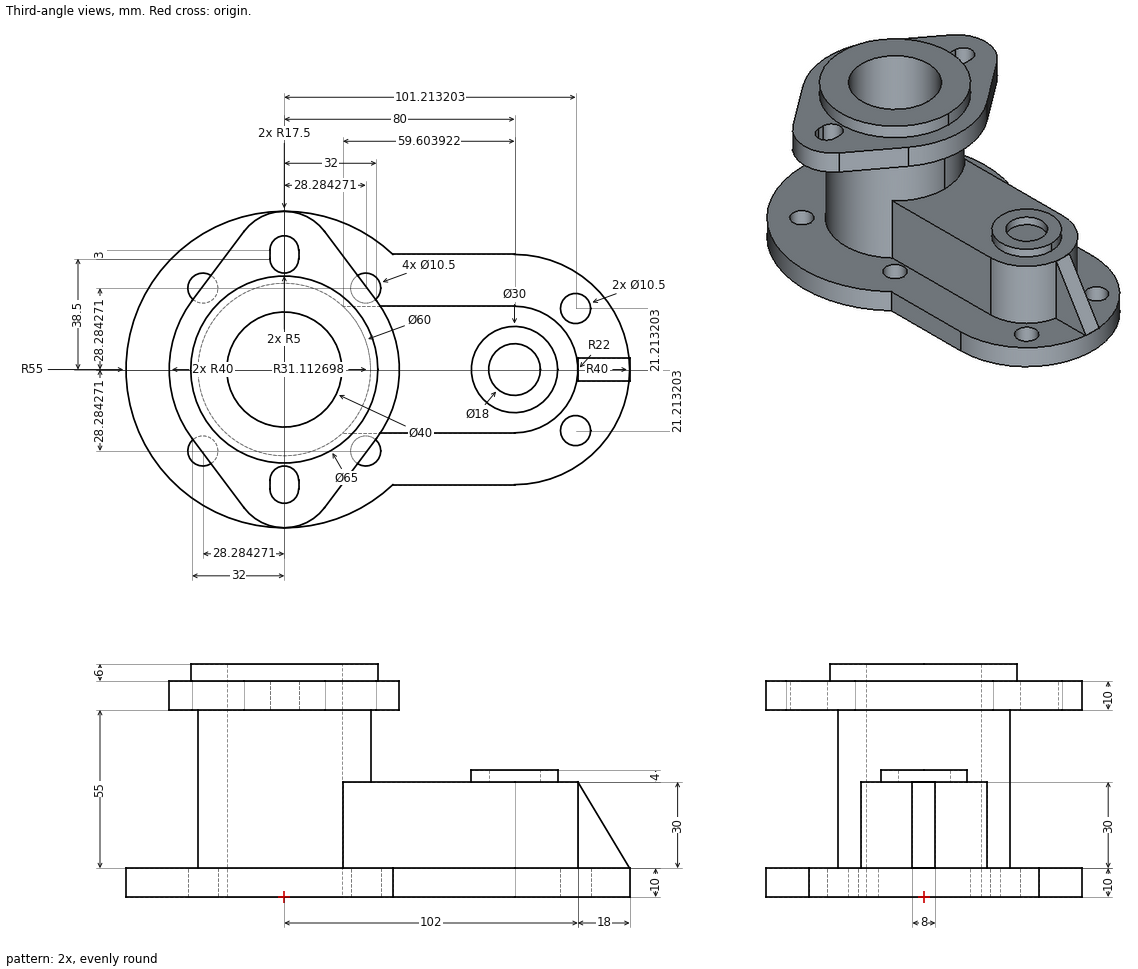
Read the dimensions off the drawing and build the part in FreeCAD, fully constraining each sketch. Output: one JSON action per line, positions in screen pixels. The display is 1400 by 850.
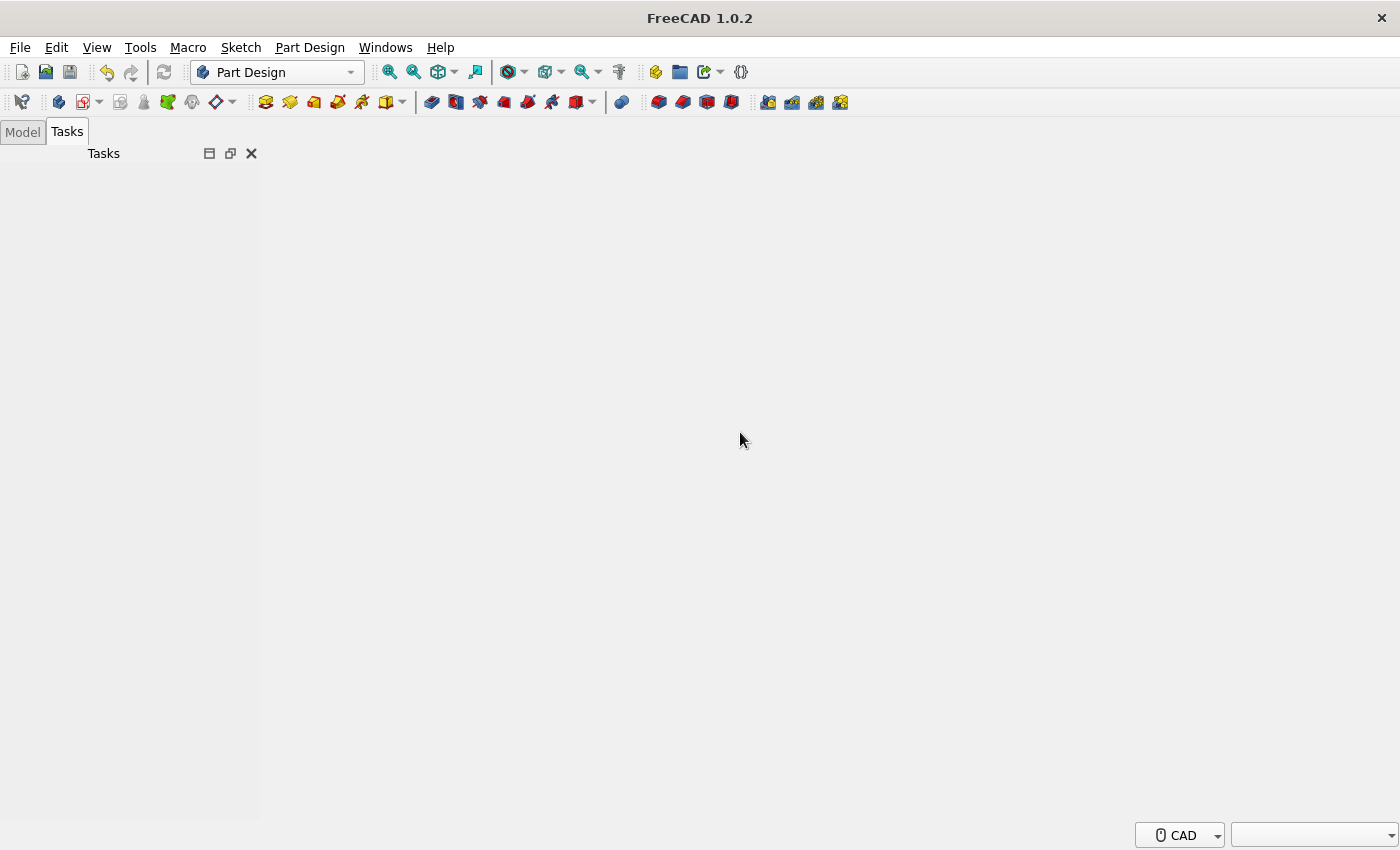
{"action": "key", "text": "ctrl+n"}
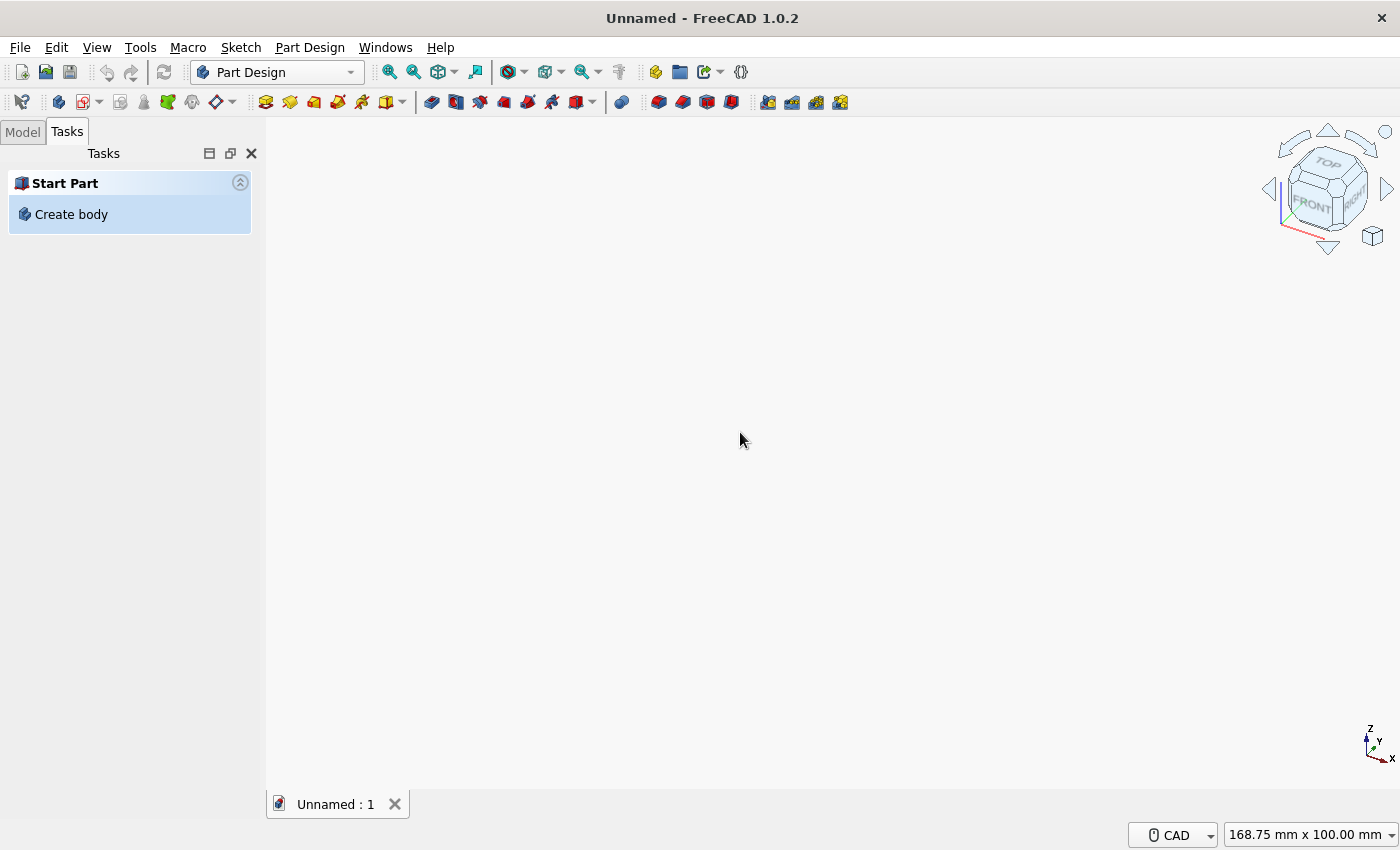
{"action": "left_click", "coordinate": [84, 102]}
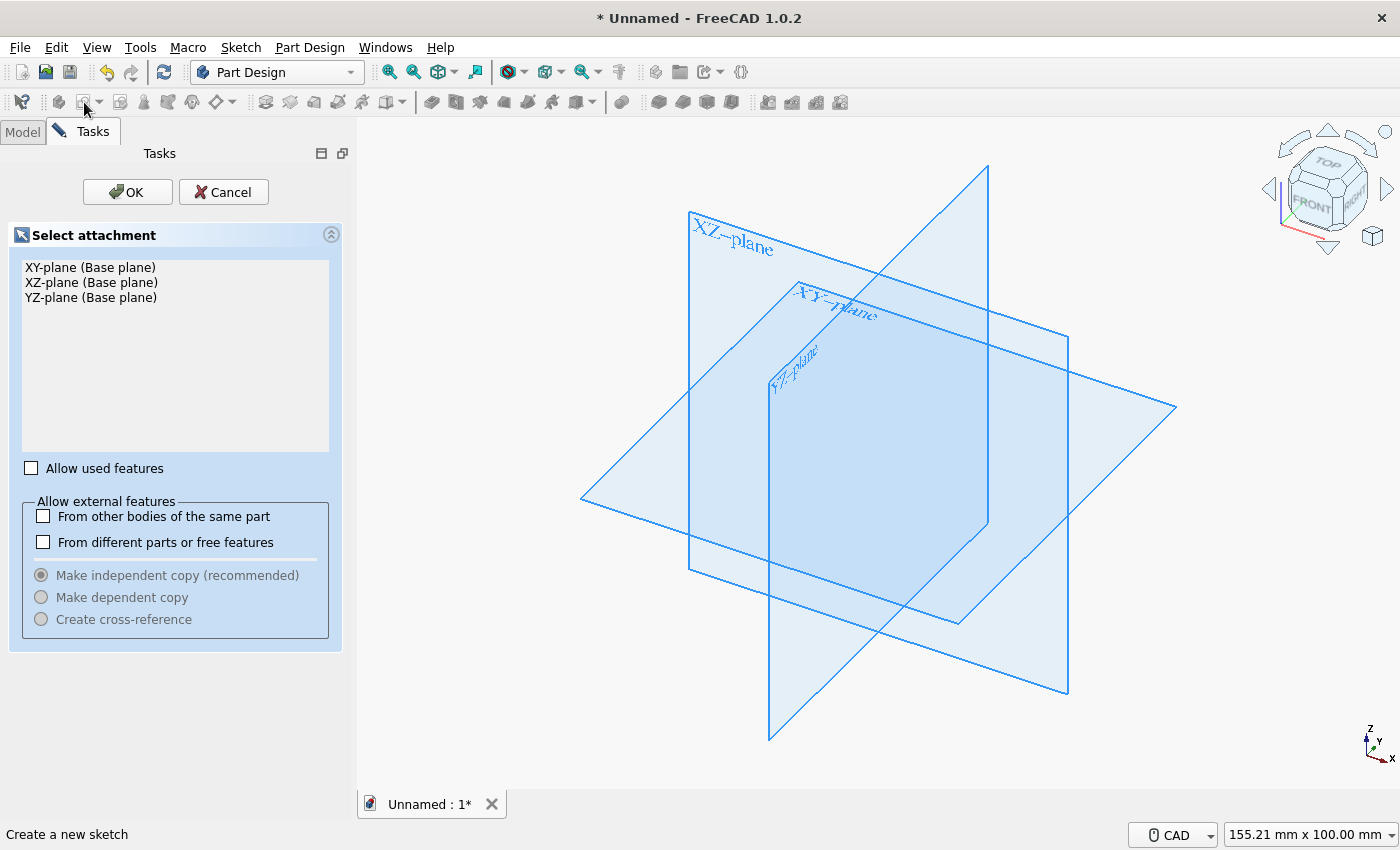
{"action": "left_click", "coordinate": [82, 268]}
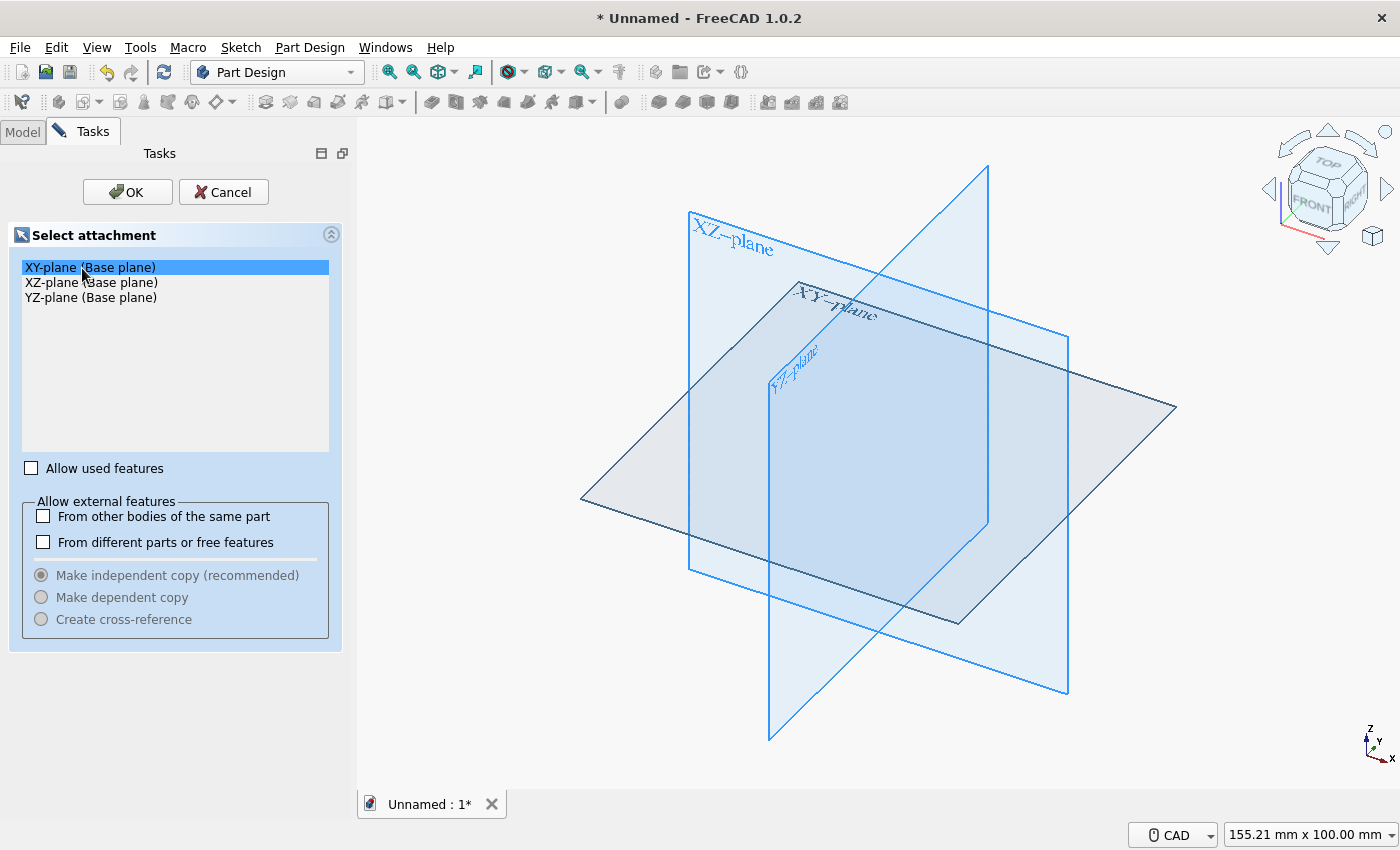
{"action": "left_click", "coordinate": [128, 192]}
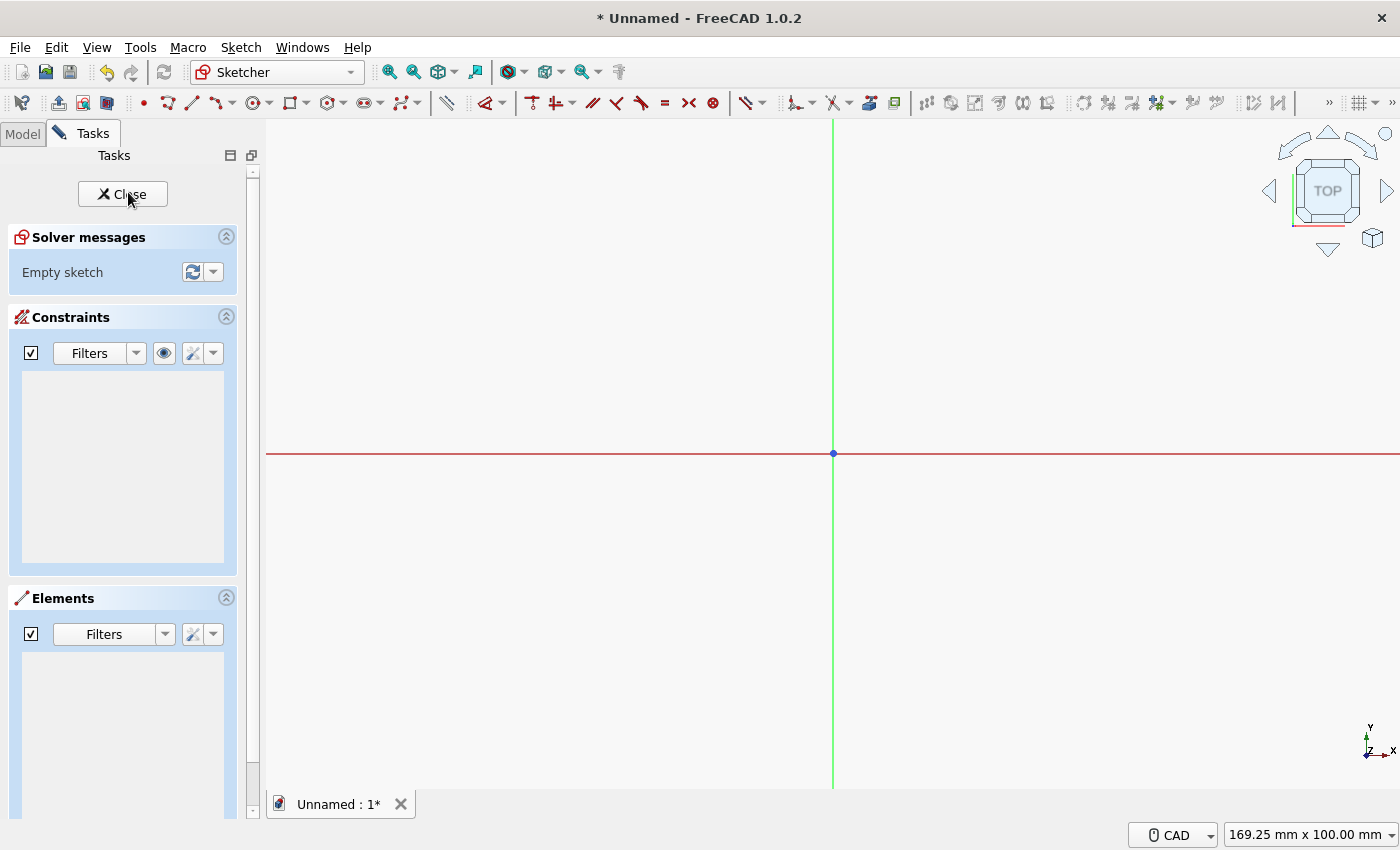
{"action": "scroll", "coordinate": [416, 454], "scroll_direction": "down", "scroll_amount": 3}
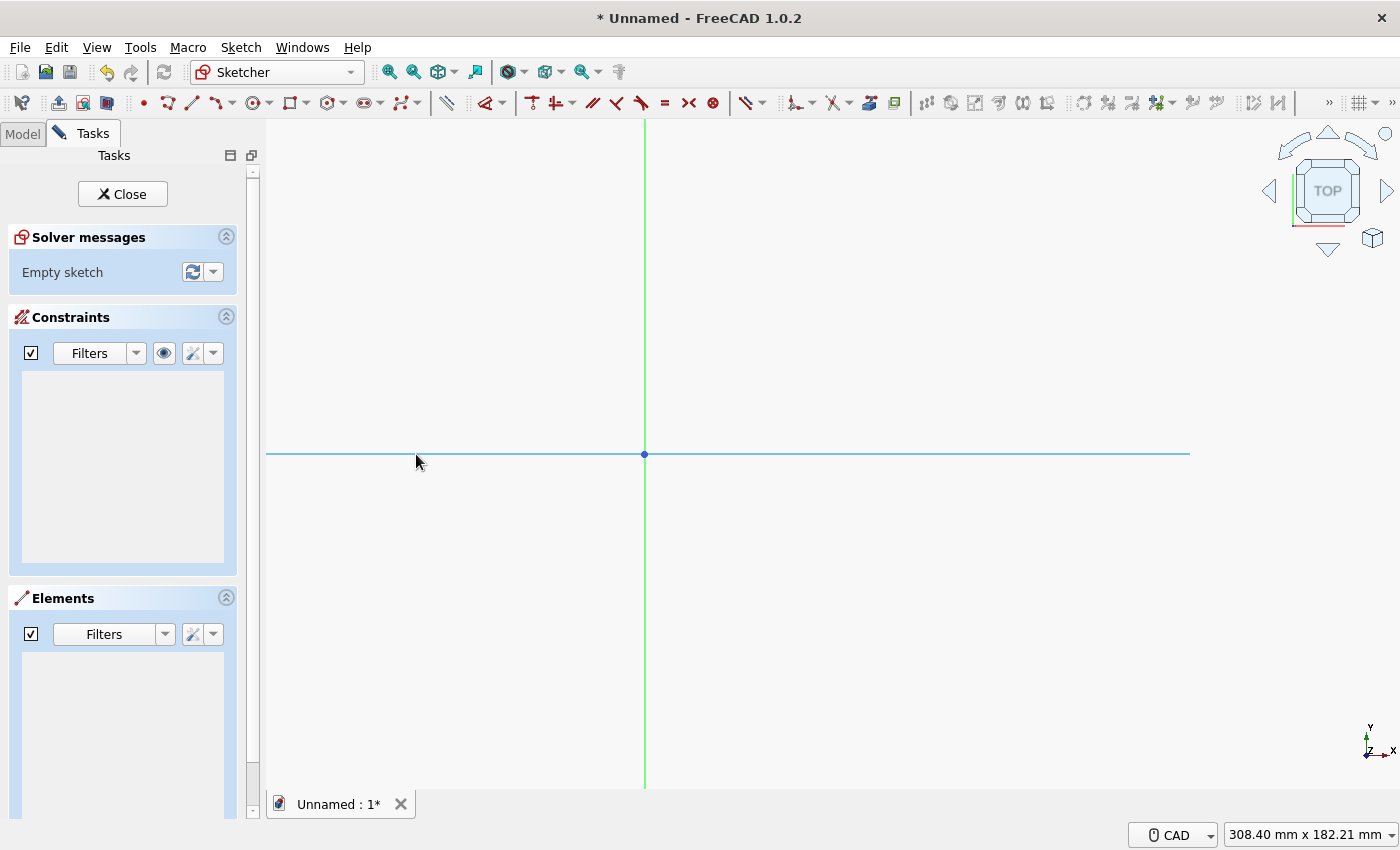
{"action": "left_click", "coordinate": [192, 104]}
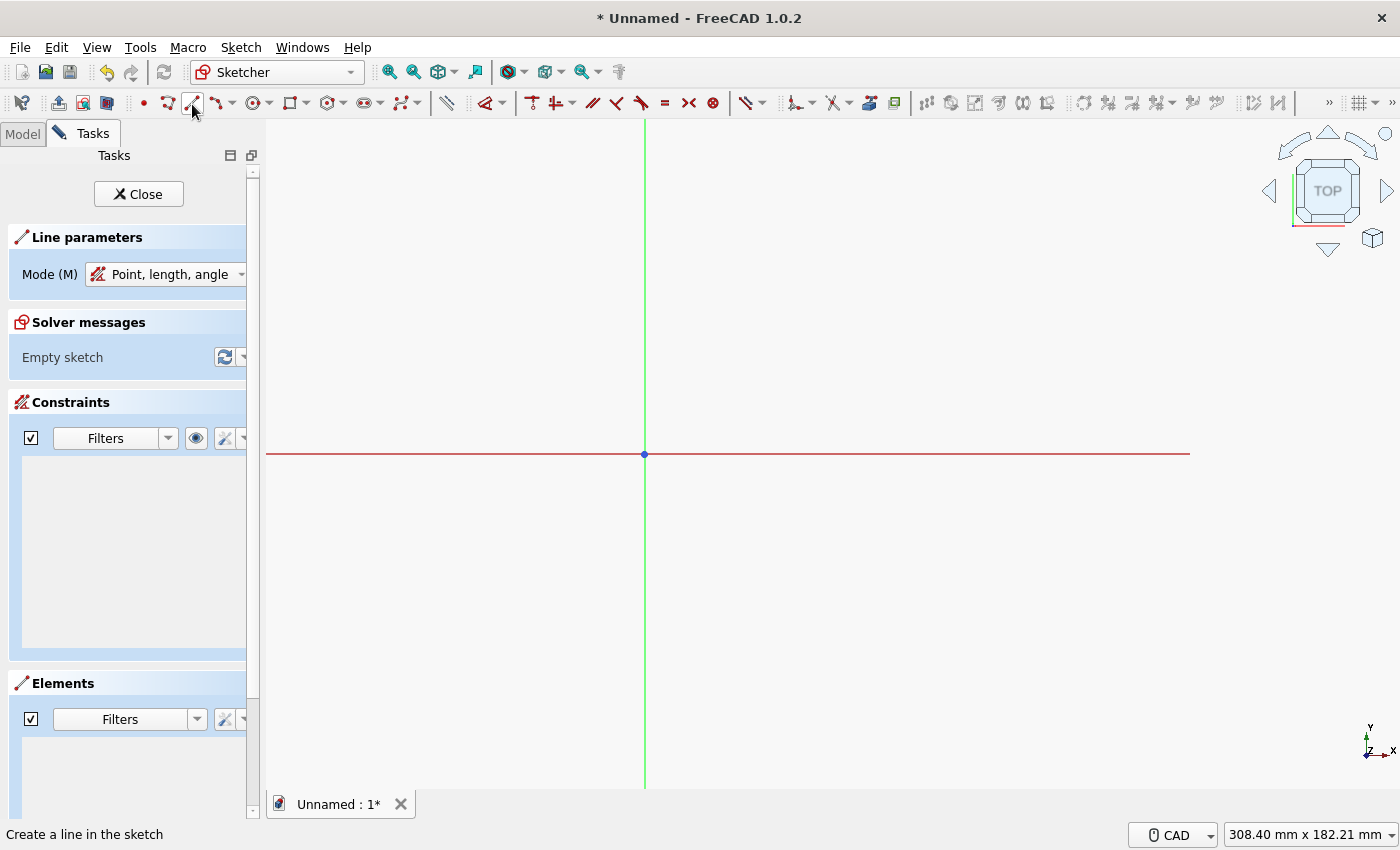
{"action": "left_click", "coordinate": [939, 307]}
{"action": "left_click", "coordinate": [784, 307]}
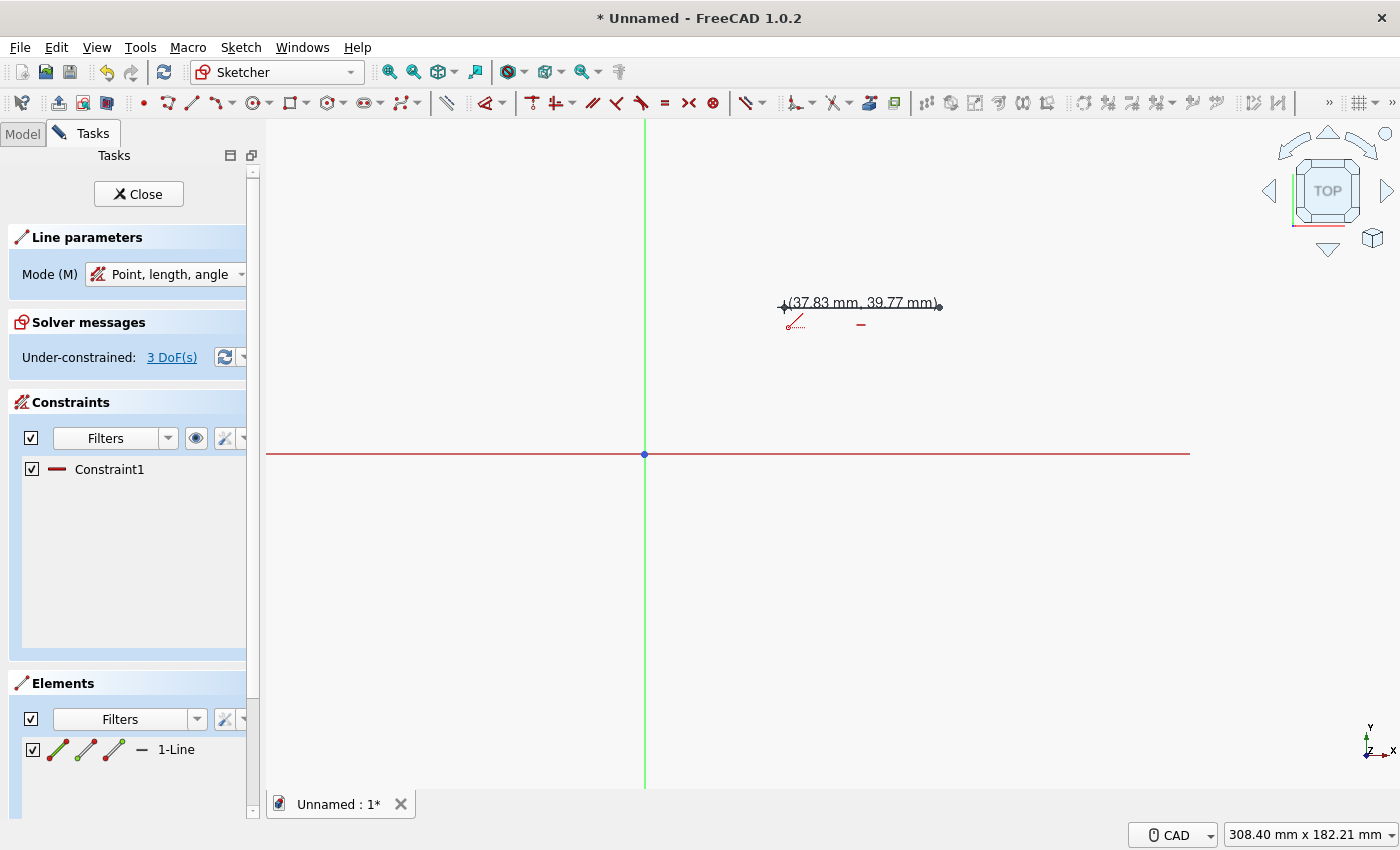
{"action": "left_click", "coordinate": [784, 601]}
{"action": "left_click", "coordinate": [939, 601]}